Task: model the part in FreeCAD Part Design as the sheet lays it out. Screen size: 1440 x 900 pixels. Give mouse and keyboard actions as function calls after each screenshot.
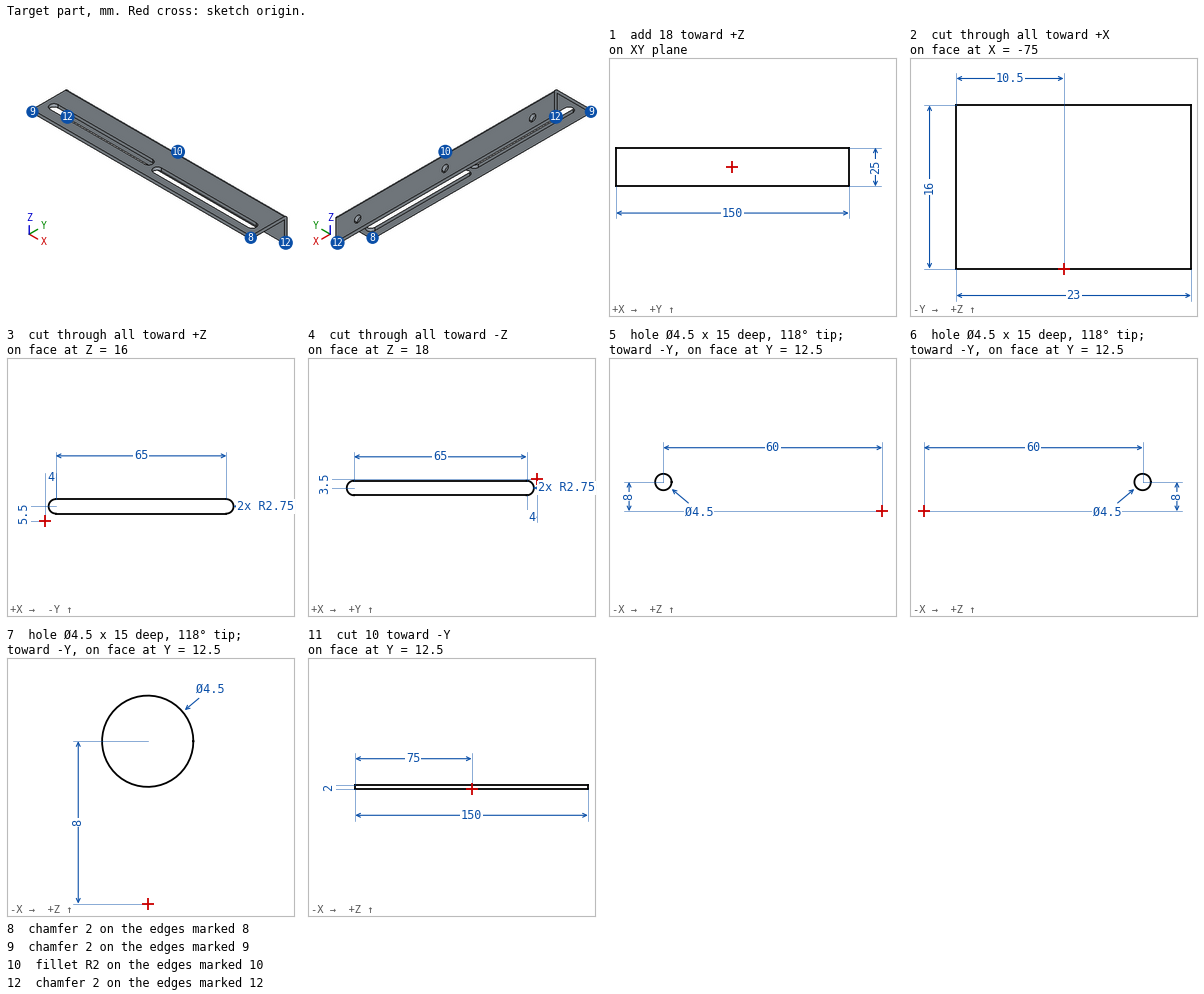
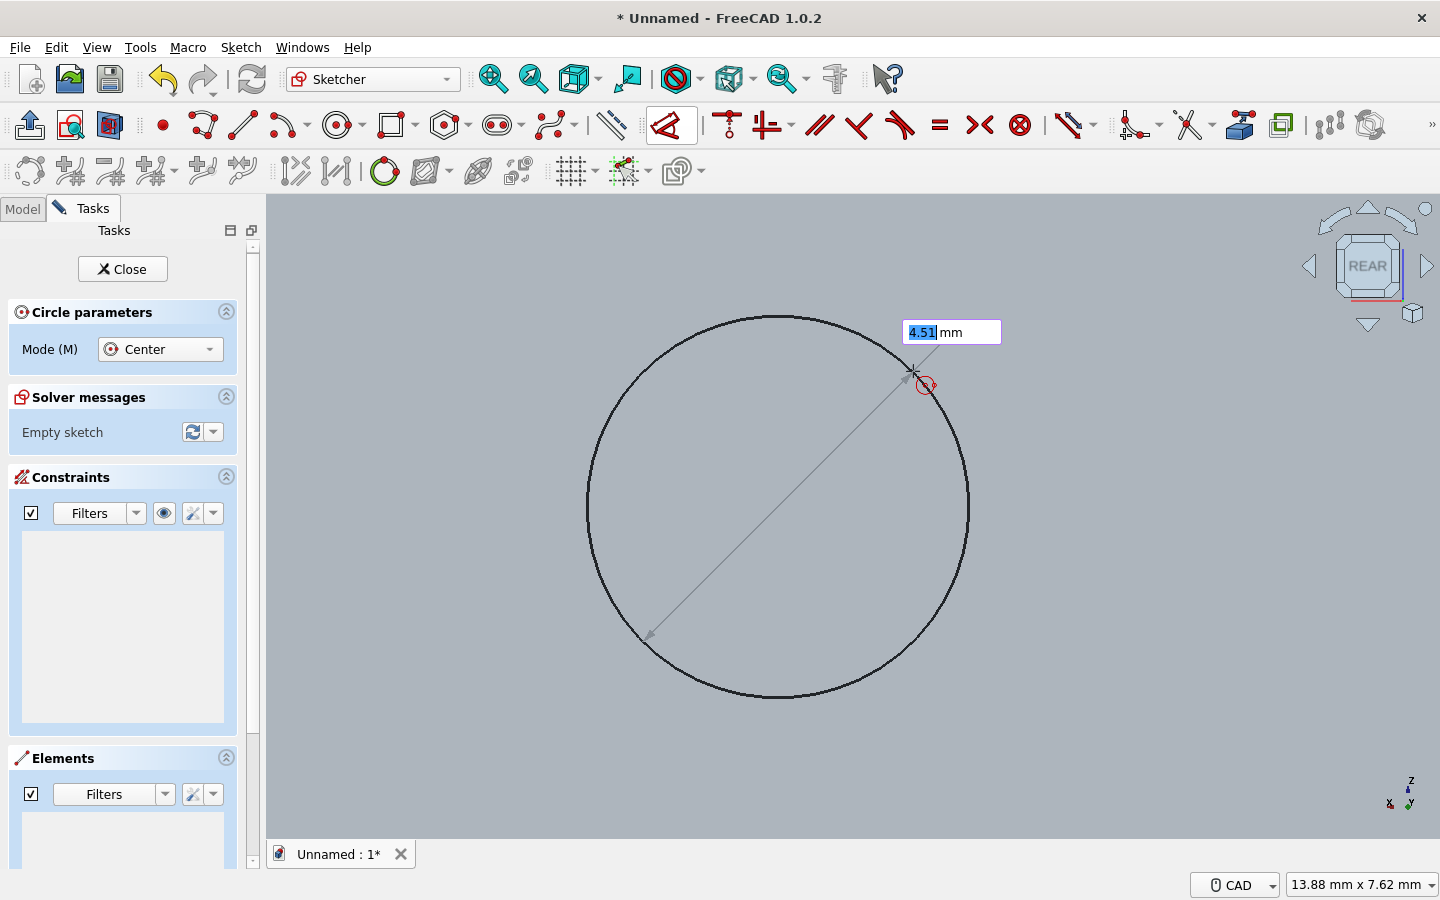
text(4.5)
key(Return)
key(Escape)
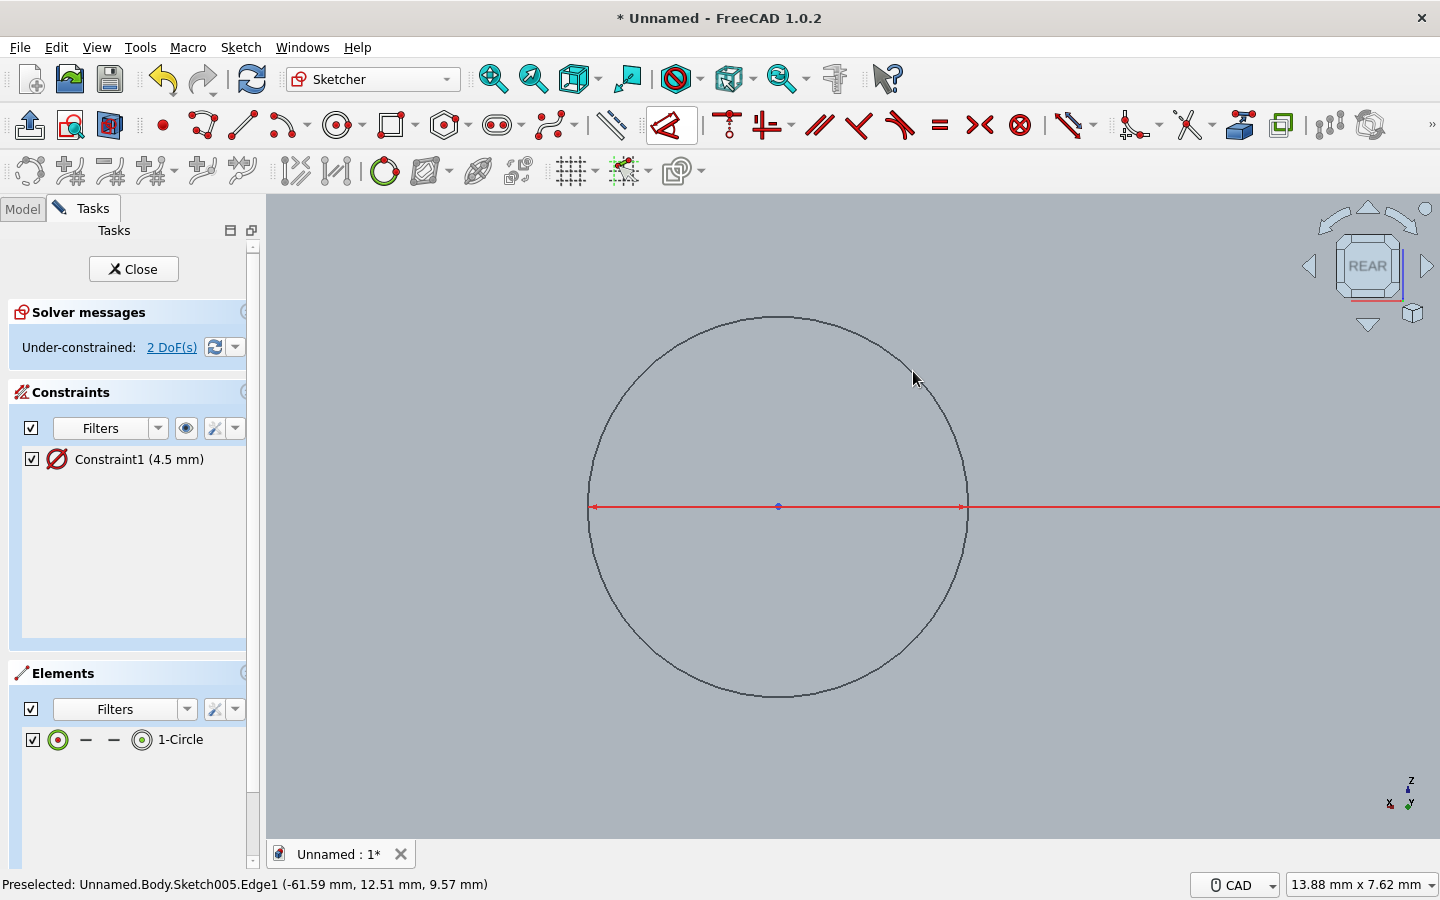
click(778, 507)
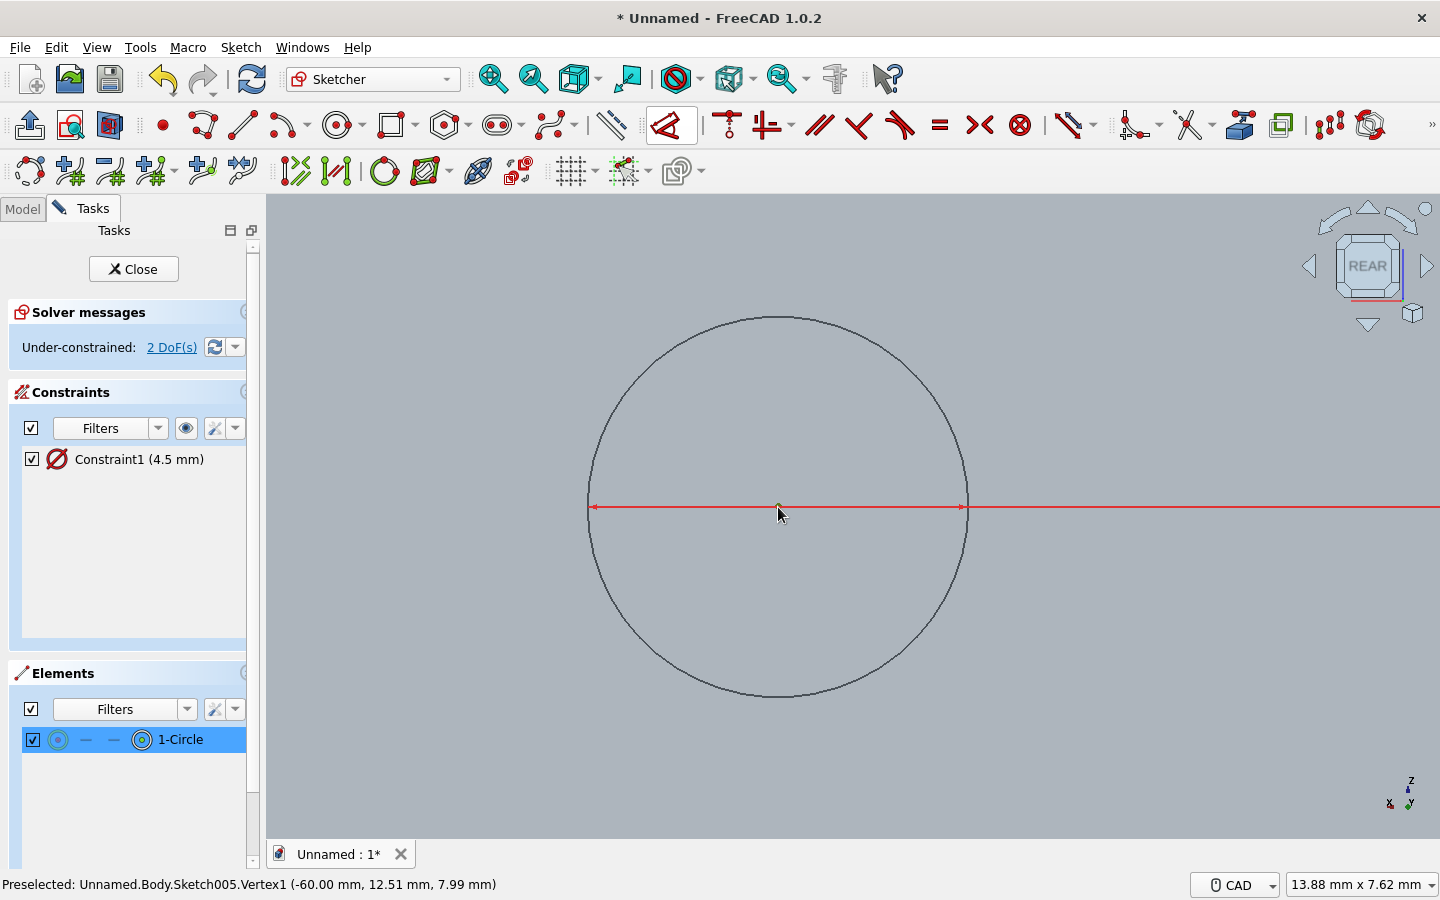
click(692, 126)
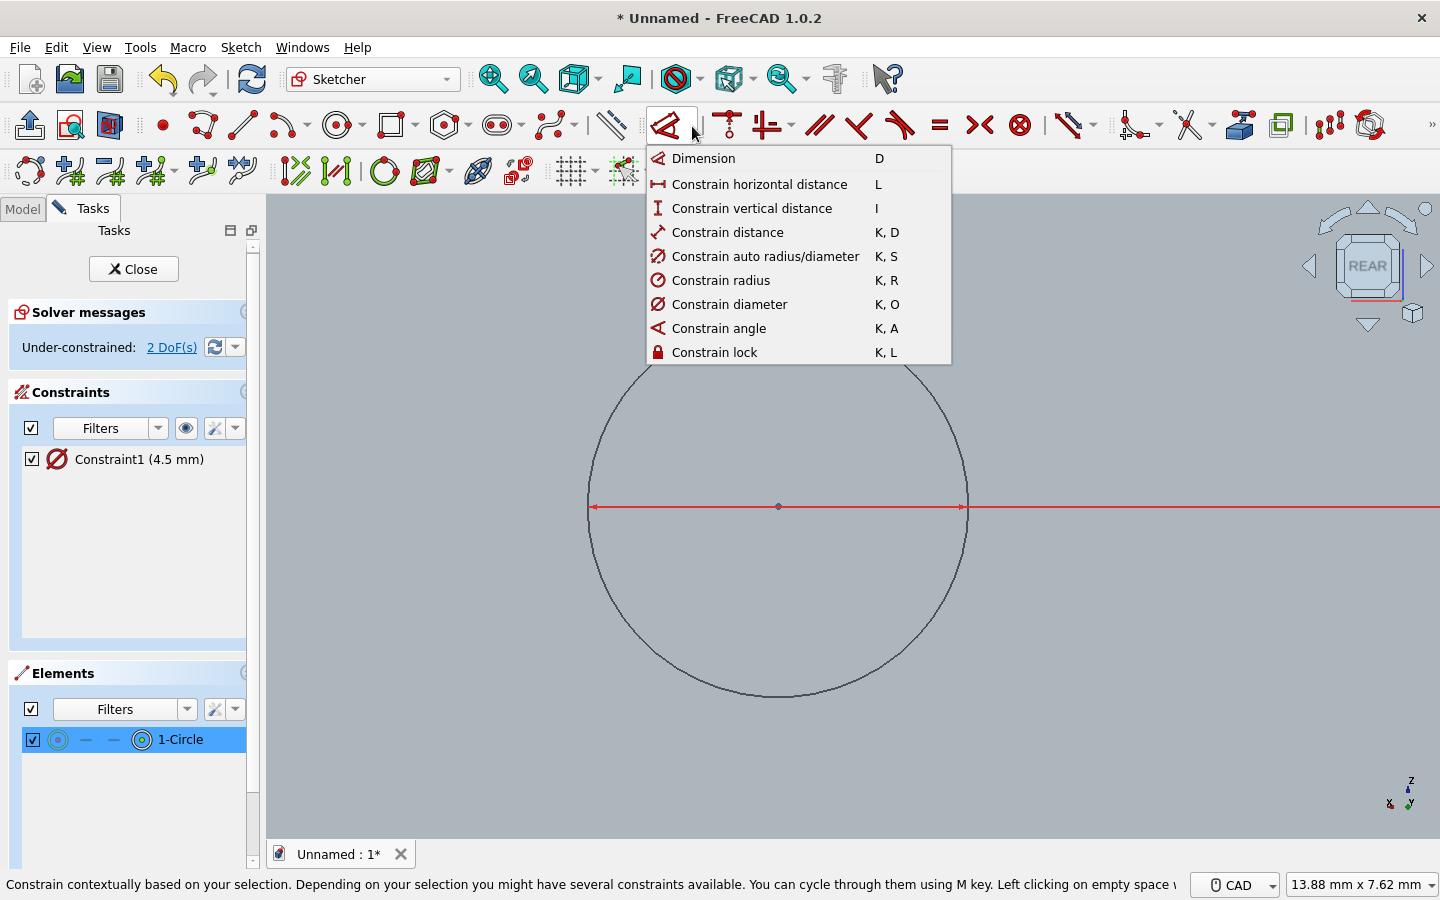
click(799, 208)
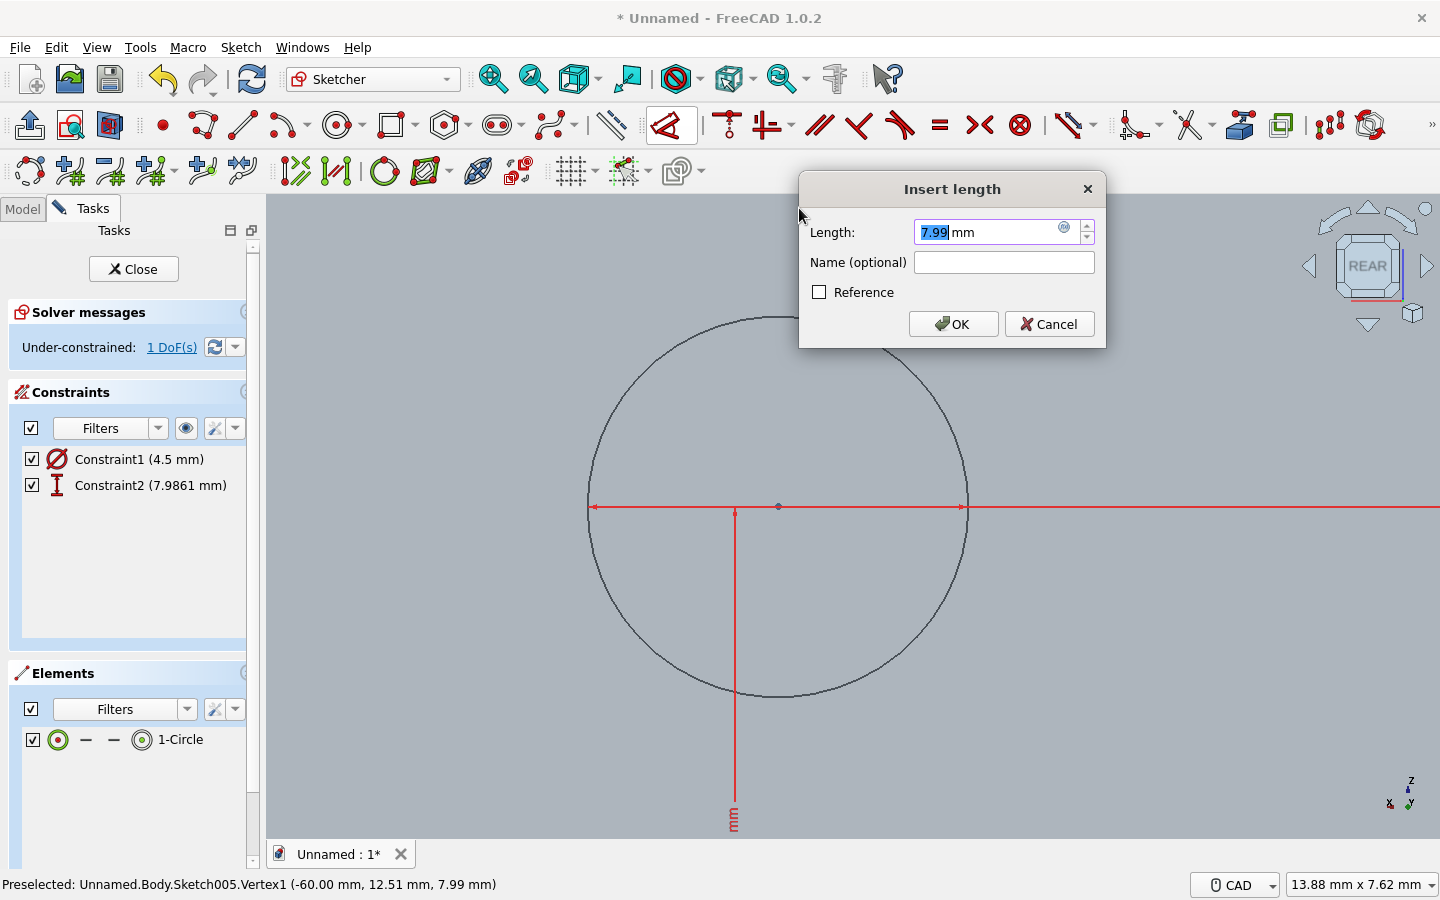
text(8)
key(Return)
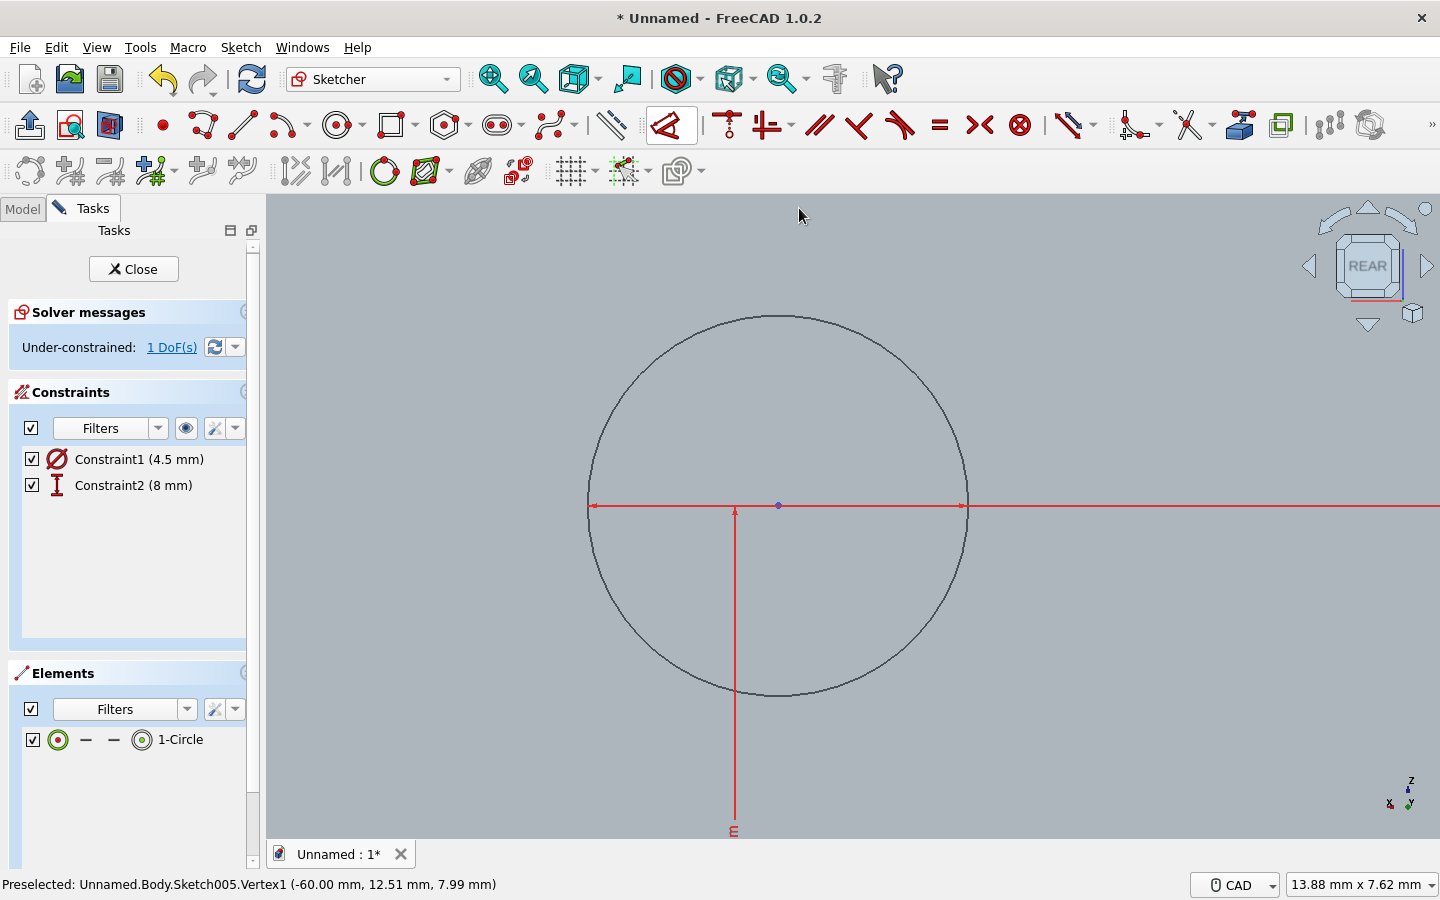
click(778, 506)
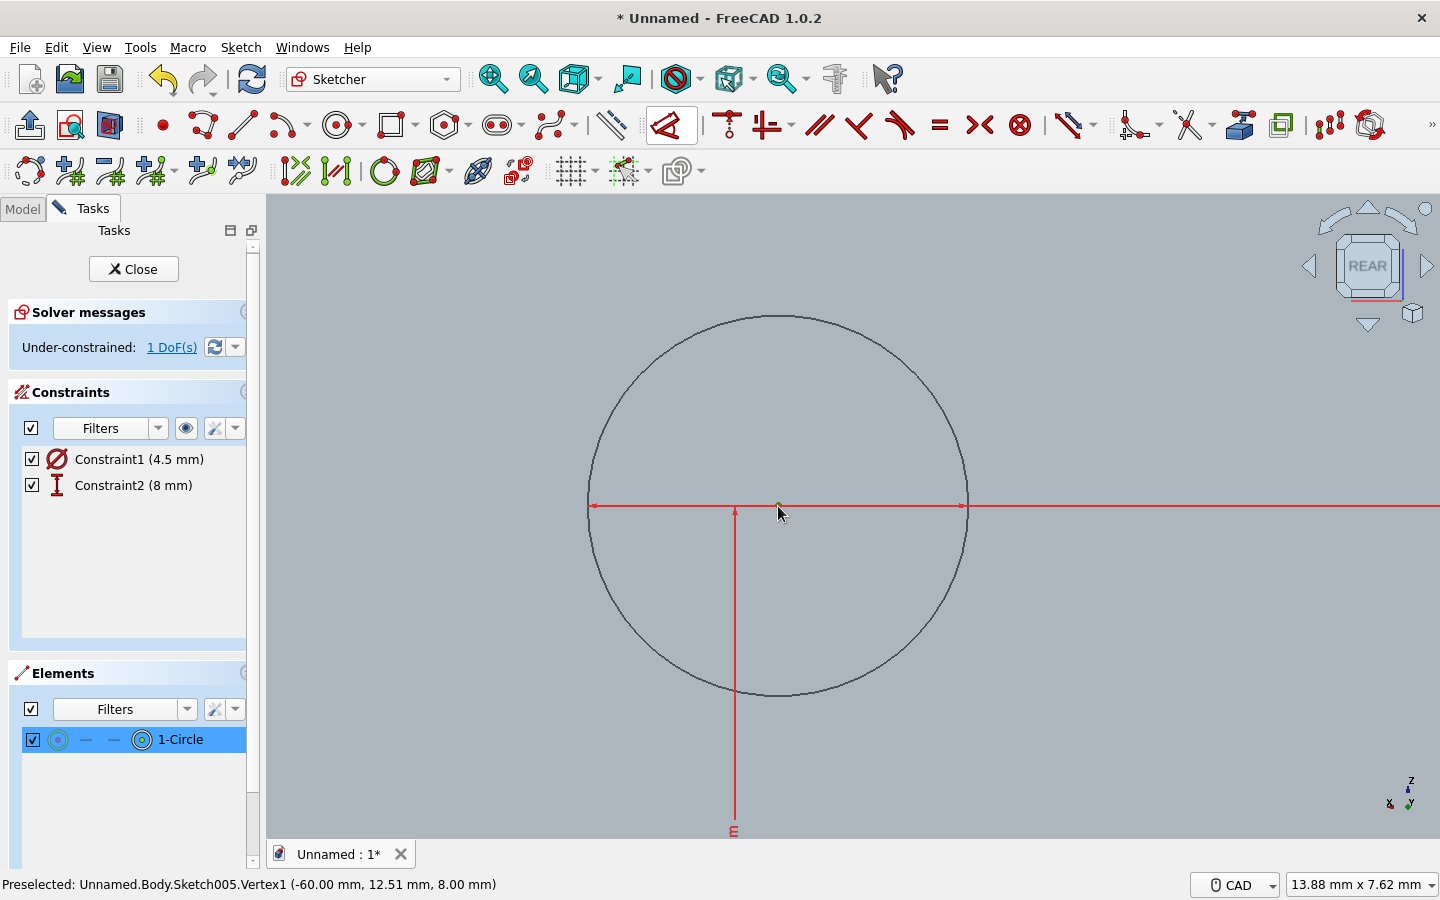
key(l)